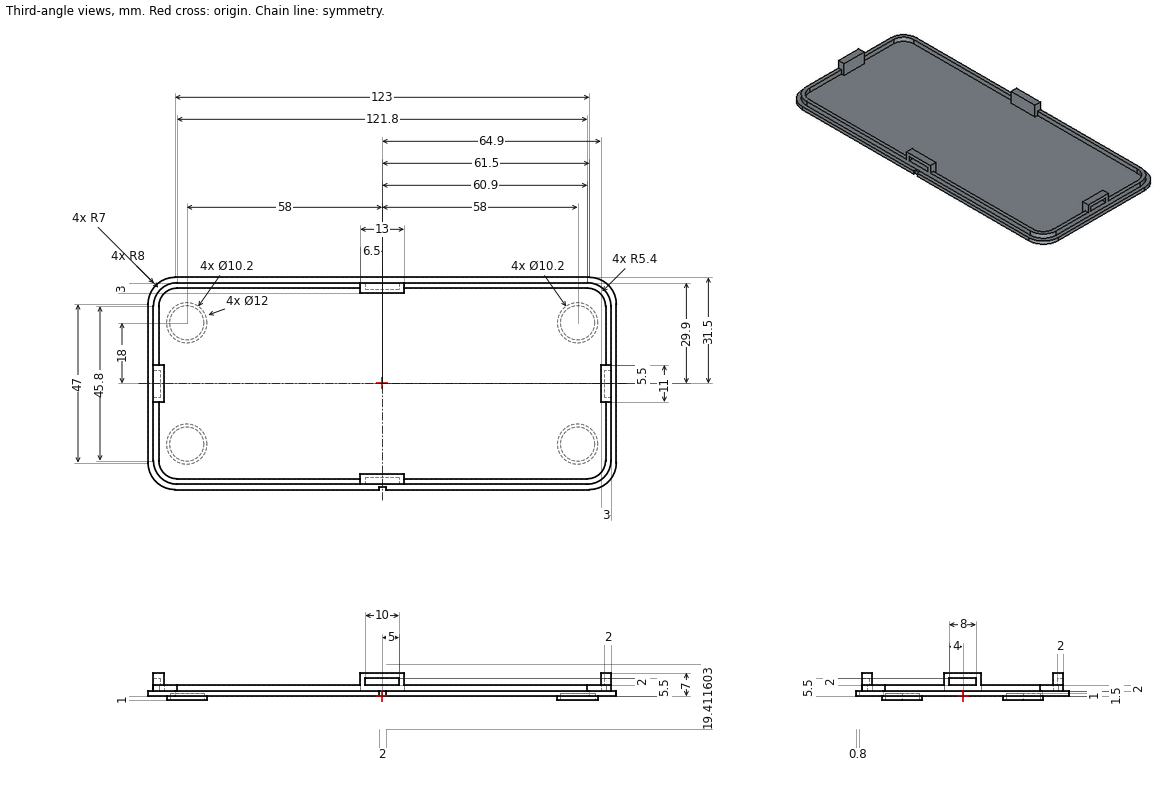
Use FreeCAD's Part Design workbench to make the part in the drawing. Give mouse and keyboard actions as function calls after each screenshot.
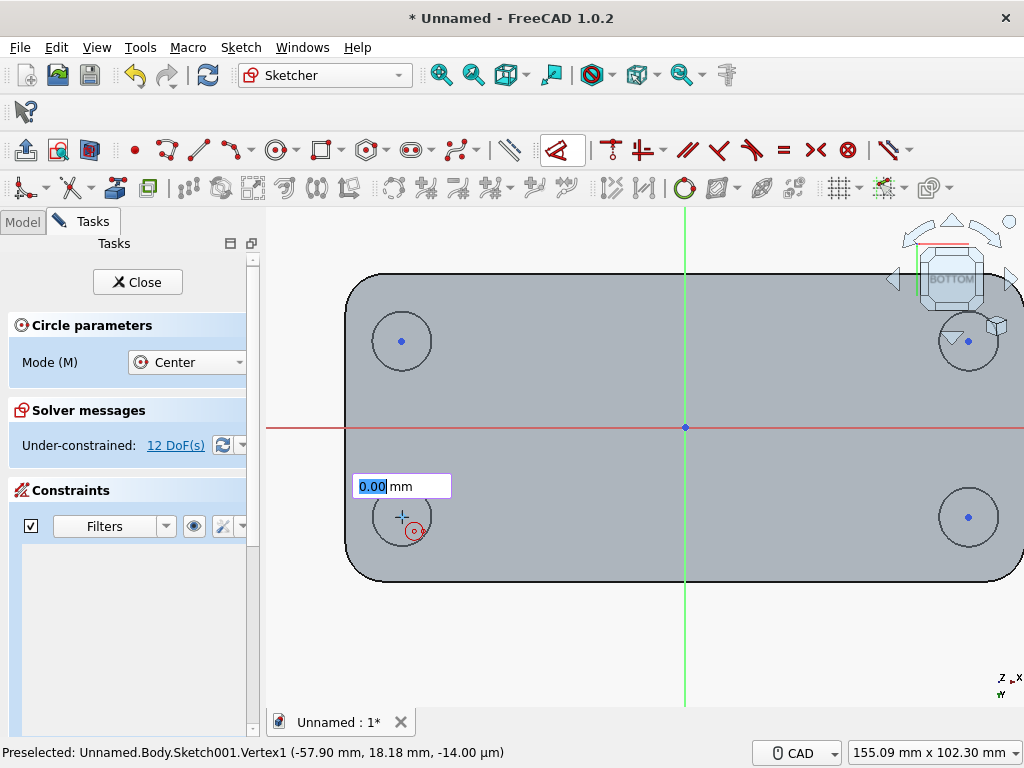
scroll(378, 507, up, 7)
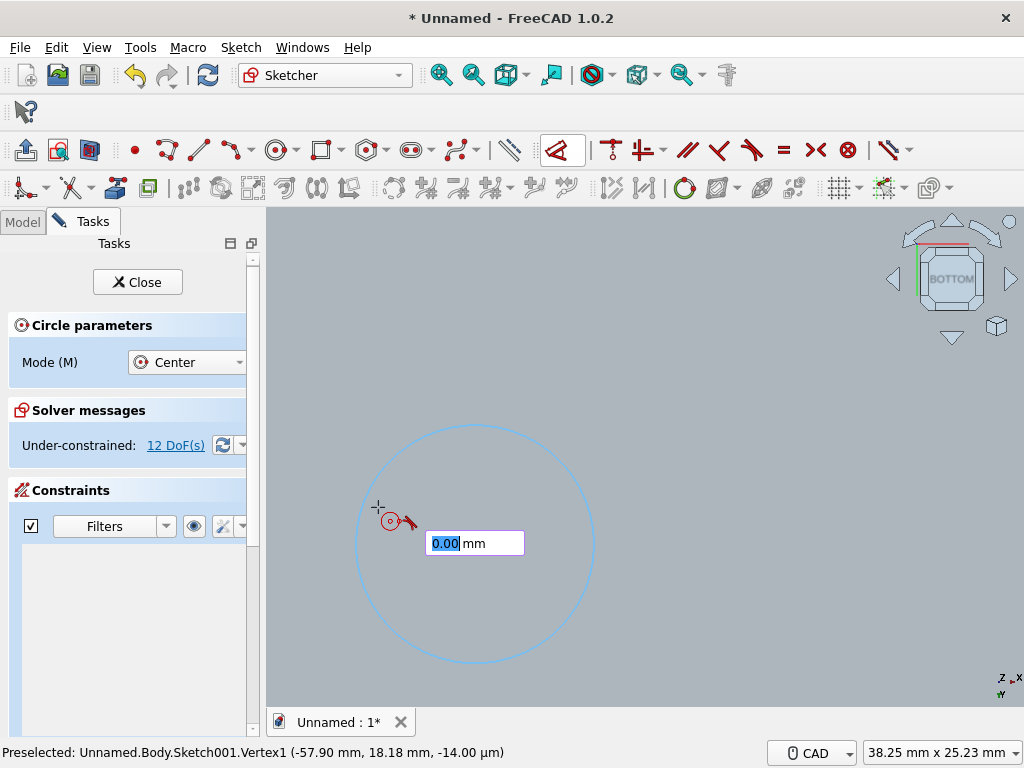
click(378, 506)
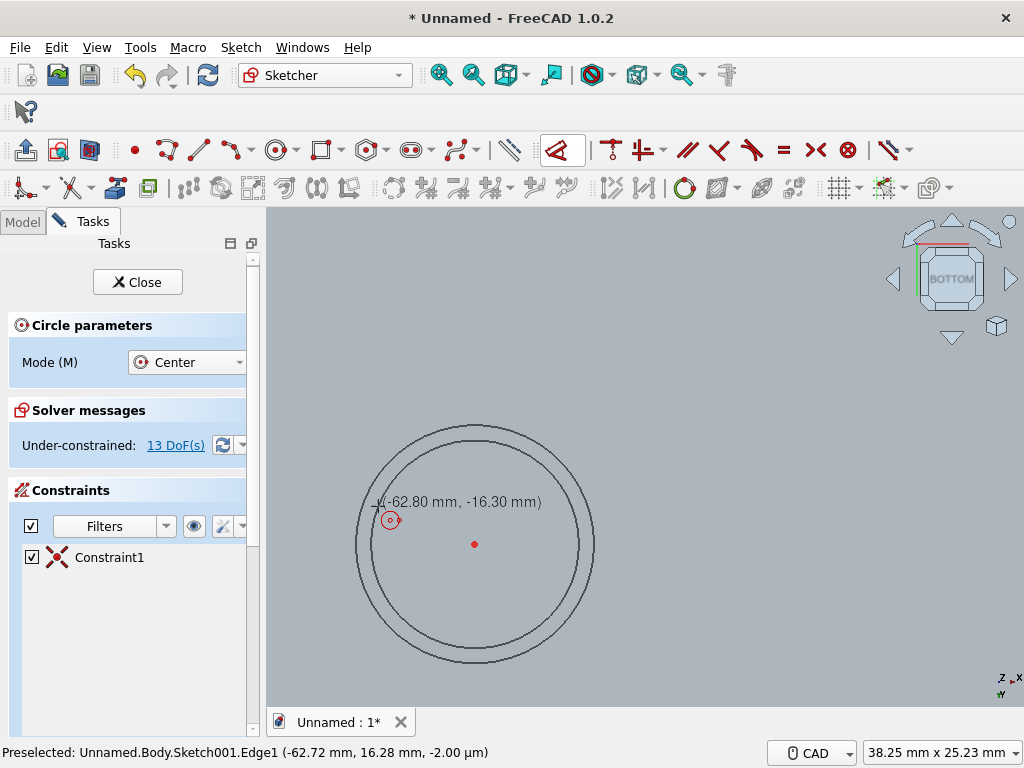
scroll(369, 511, down, 9)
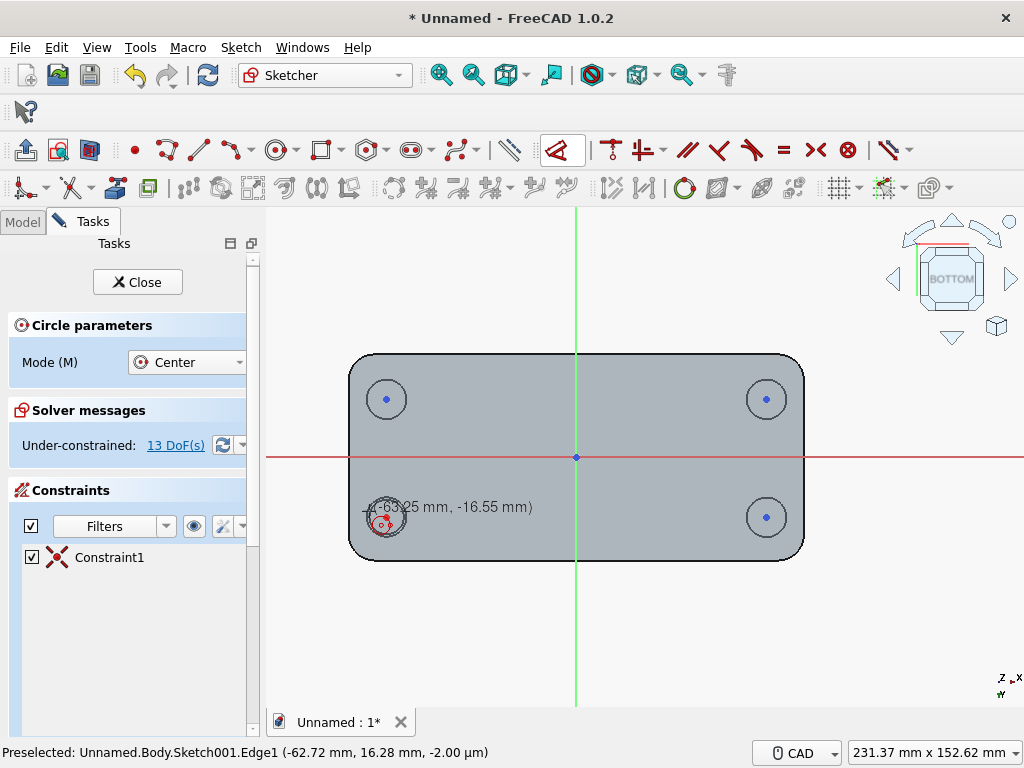
scroll(766, 516, up, 2)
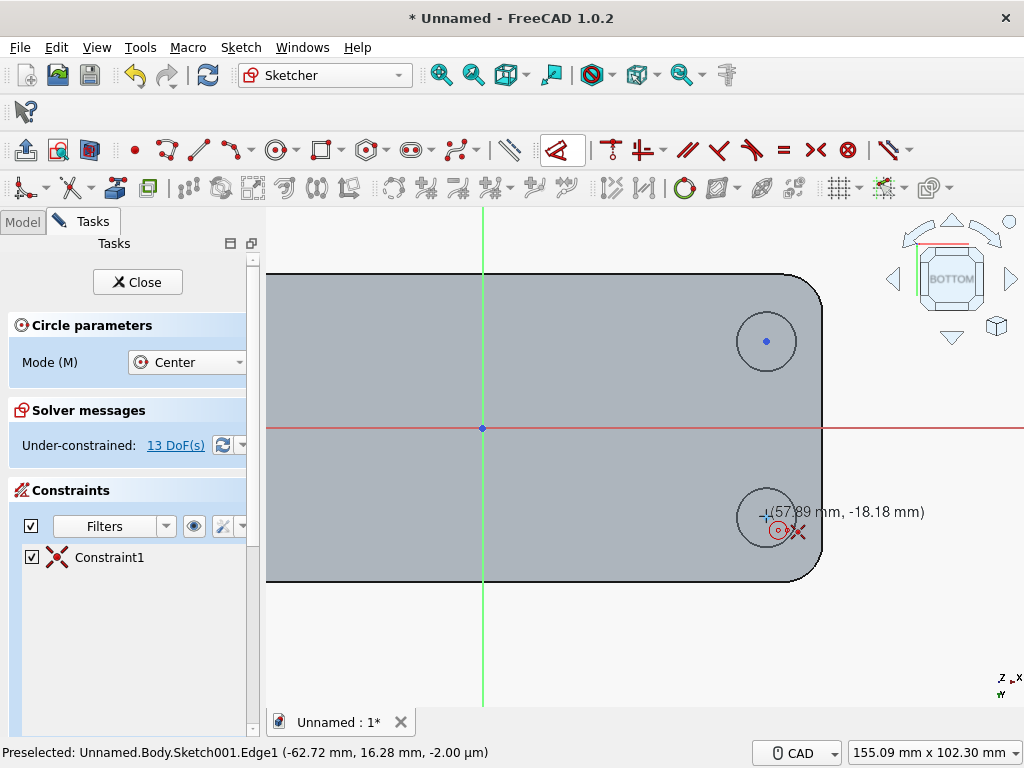
click(767, 518)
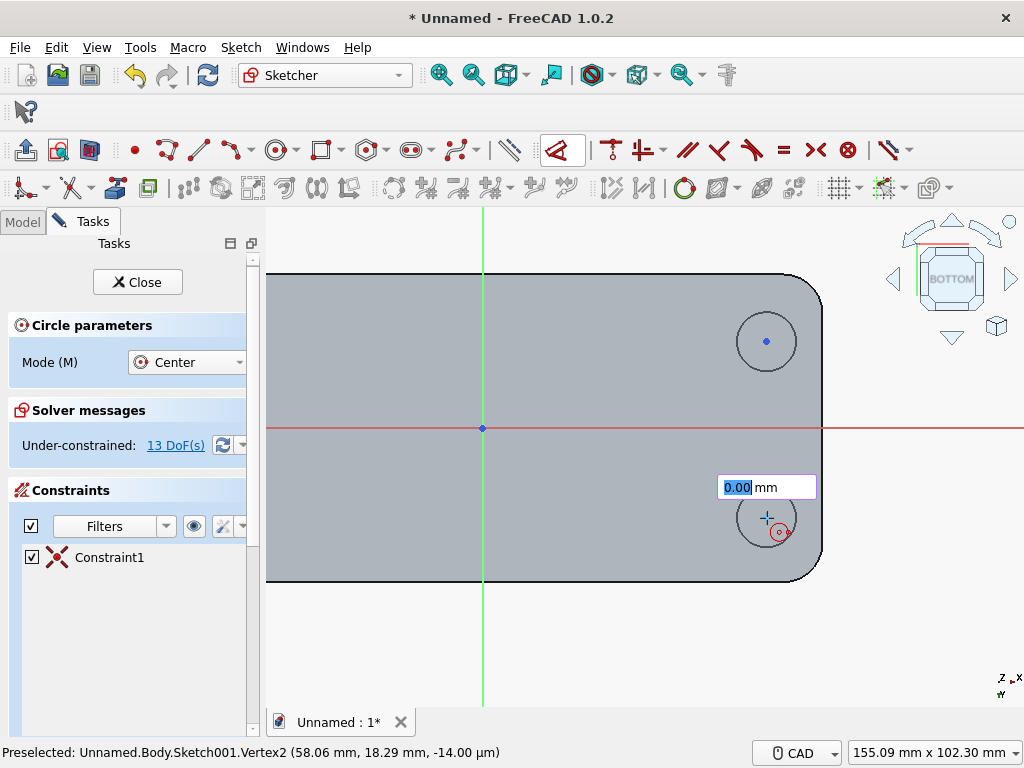
scroll(743, 508, up, 7)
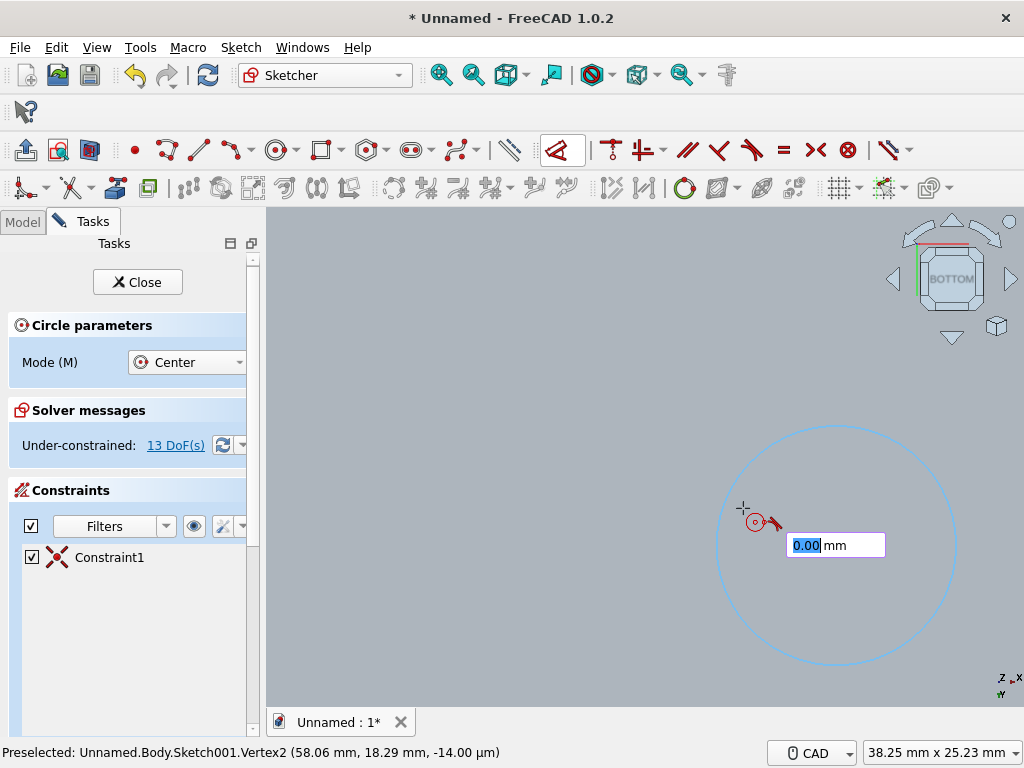
click(740, 505)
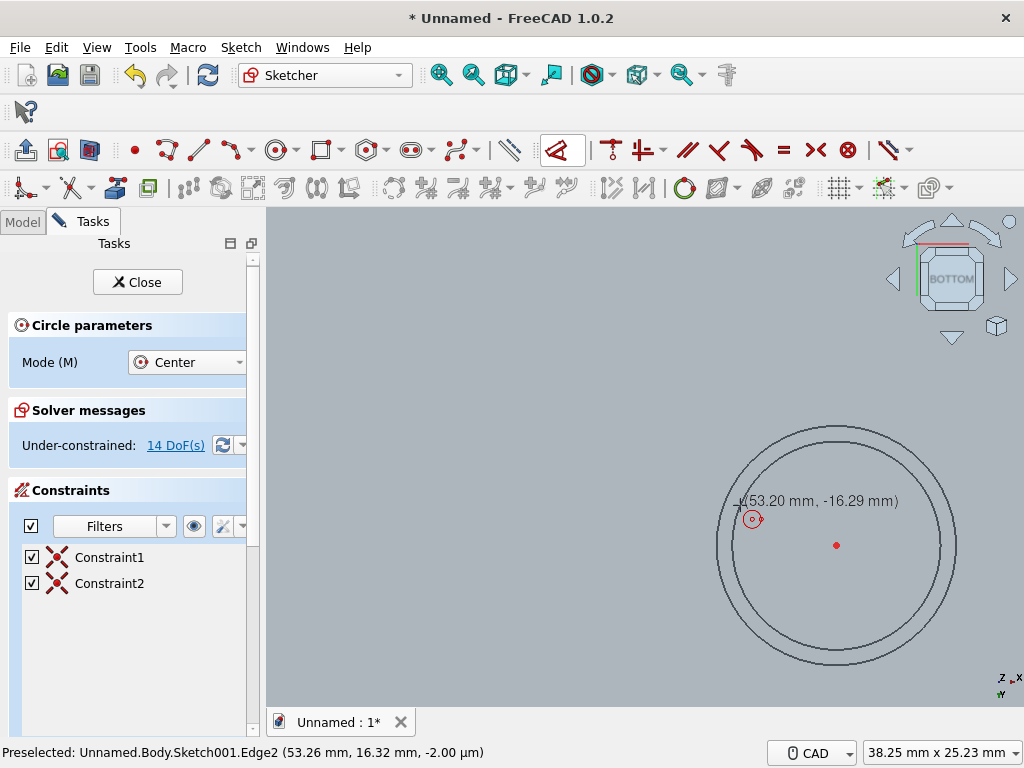
scroll(753, 511, down, 9)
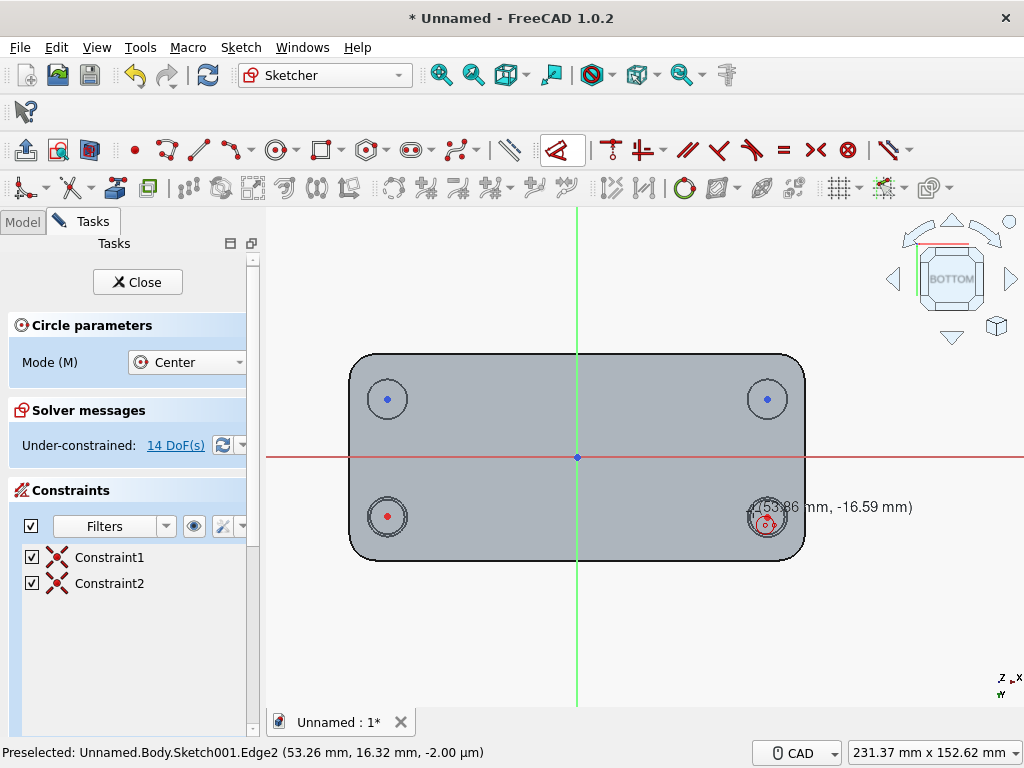
scroll(387, 398, up, 2)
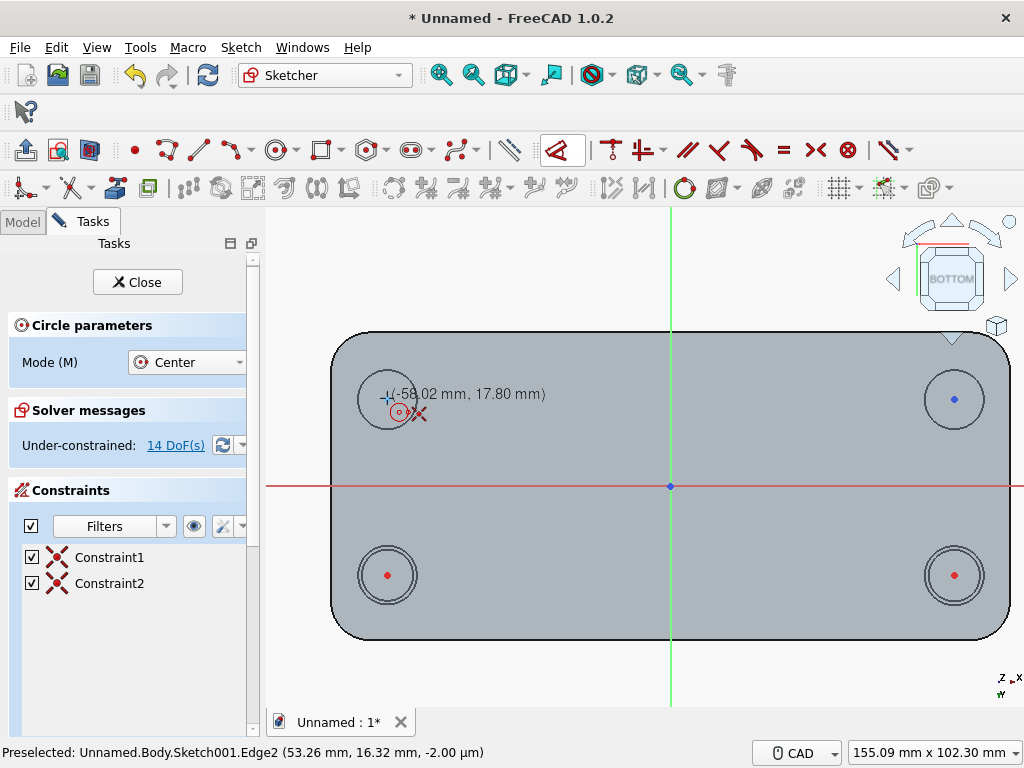
click(387, 400)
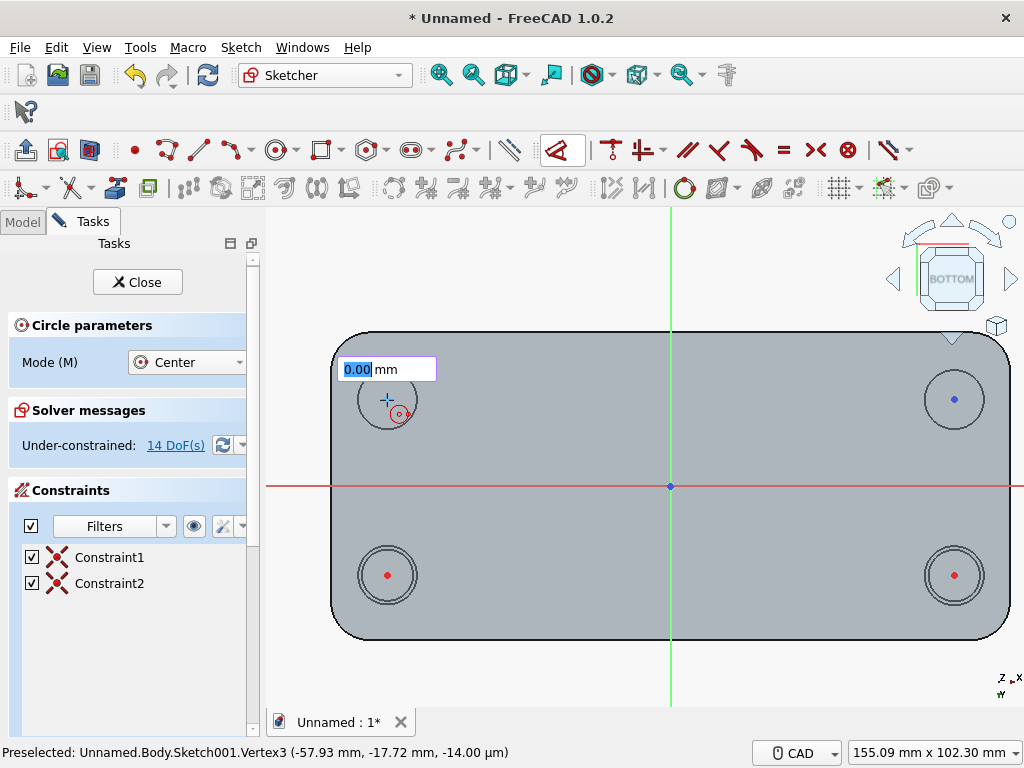
scroll(364, 390, up, 7)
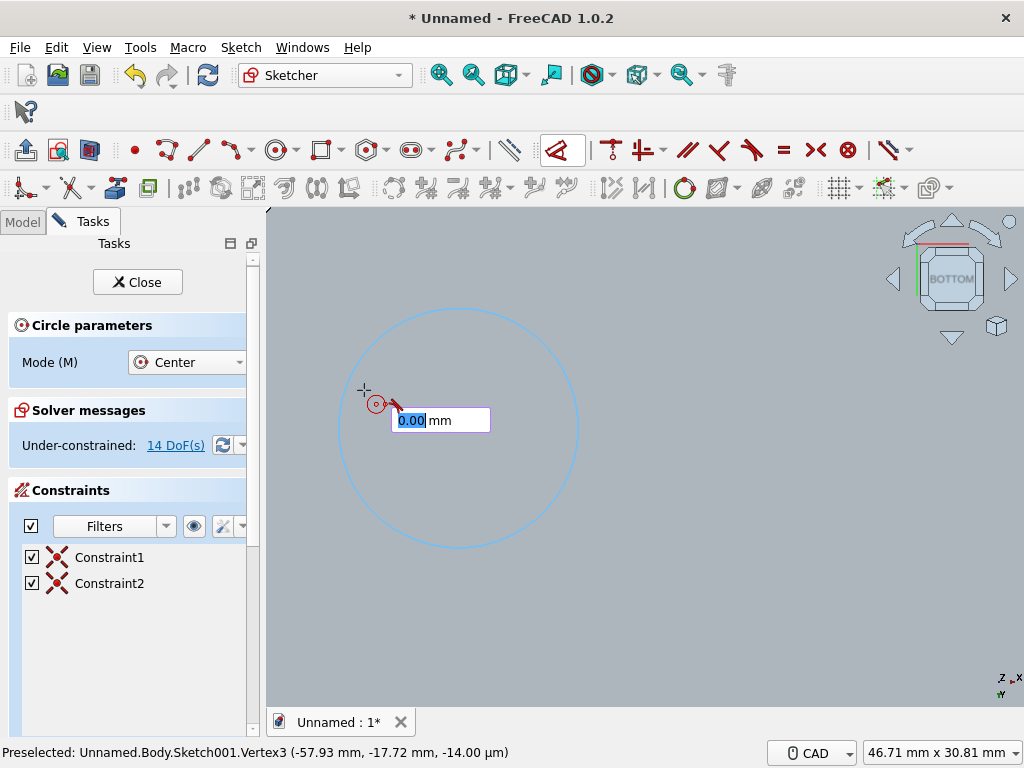
click(362, 388)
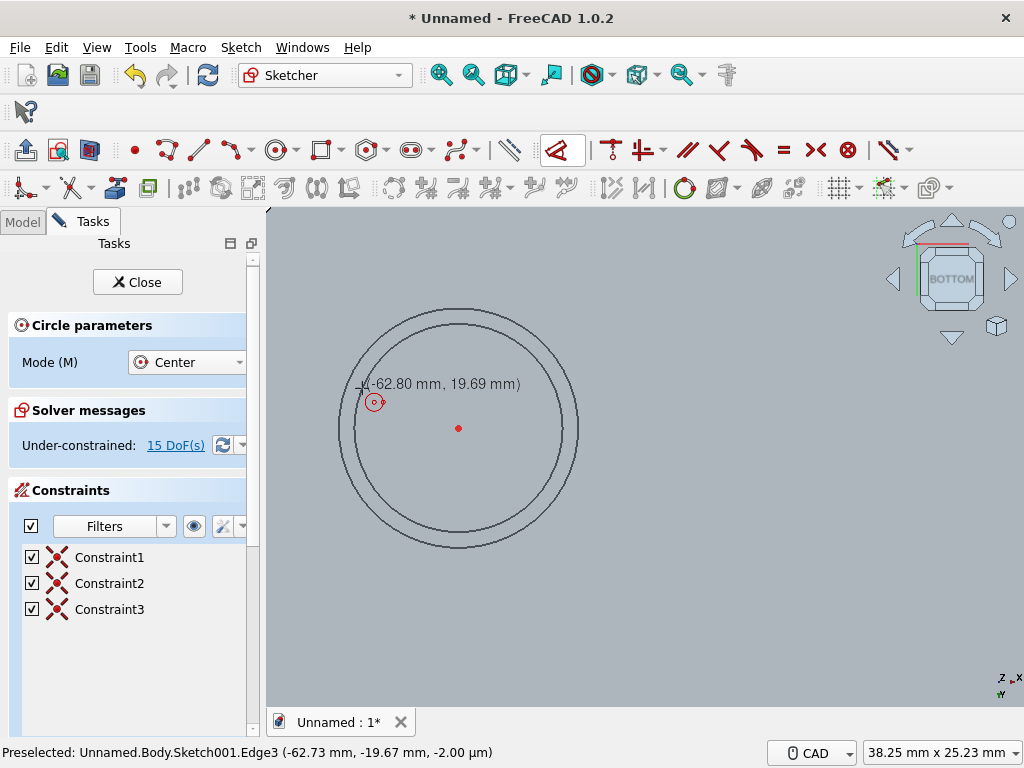
scroll(373, 393, down, 9)